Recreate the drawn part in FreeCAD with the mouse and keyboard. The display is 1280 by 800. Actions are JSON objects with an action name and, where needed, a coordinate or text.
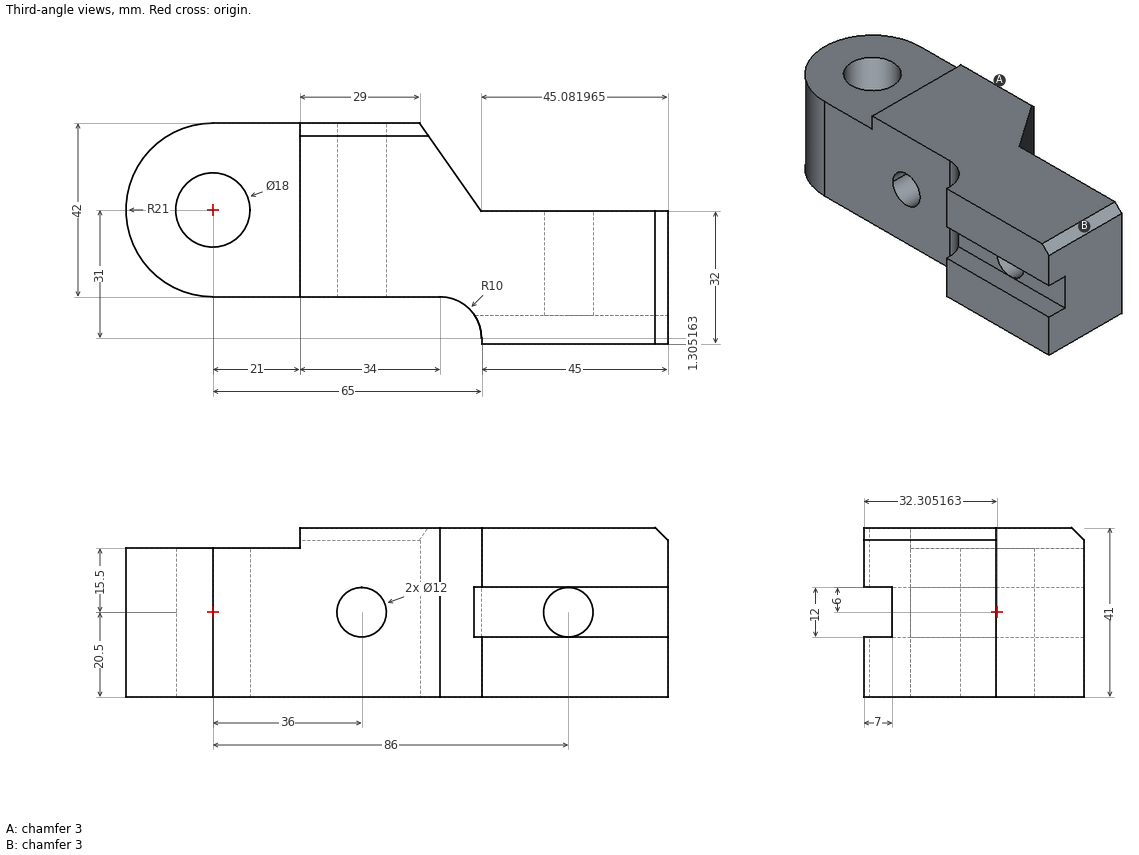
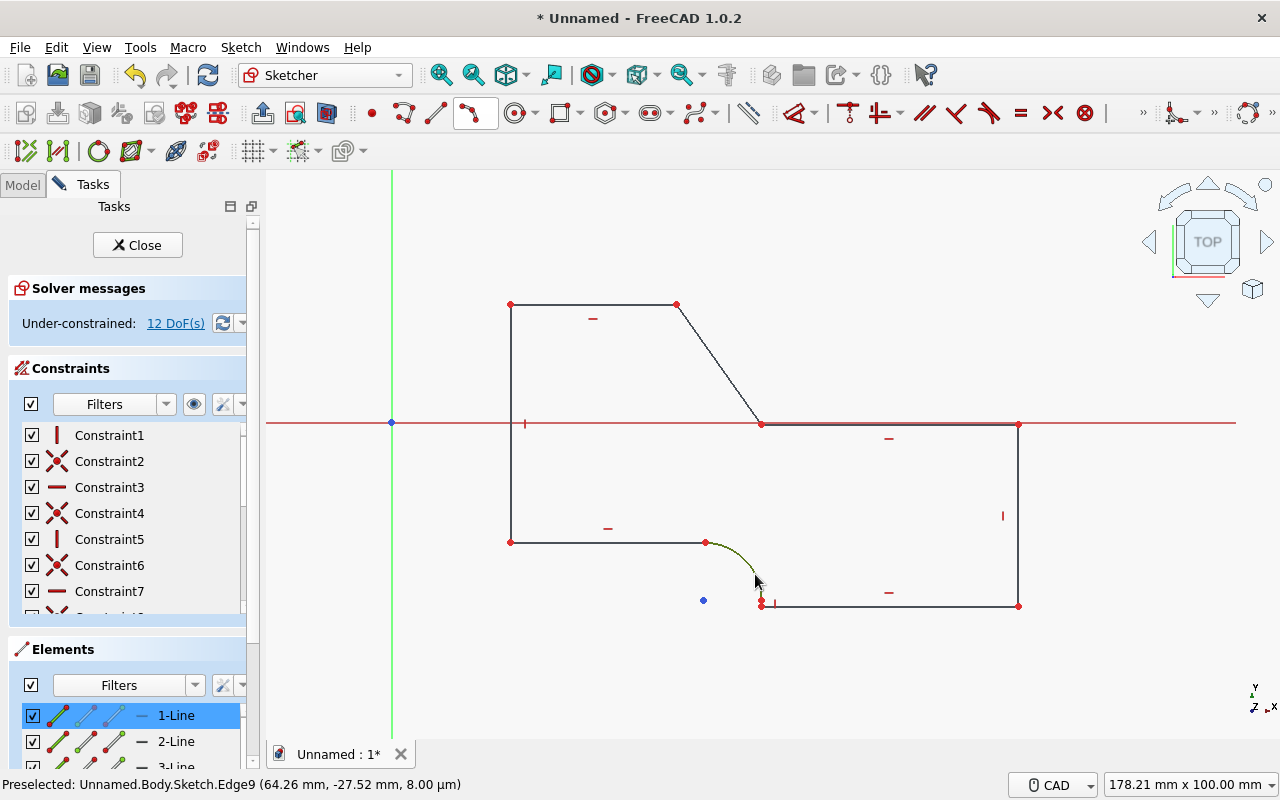
{"action": "left_click", "coordinate": [990, 114]}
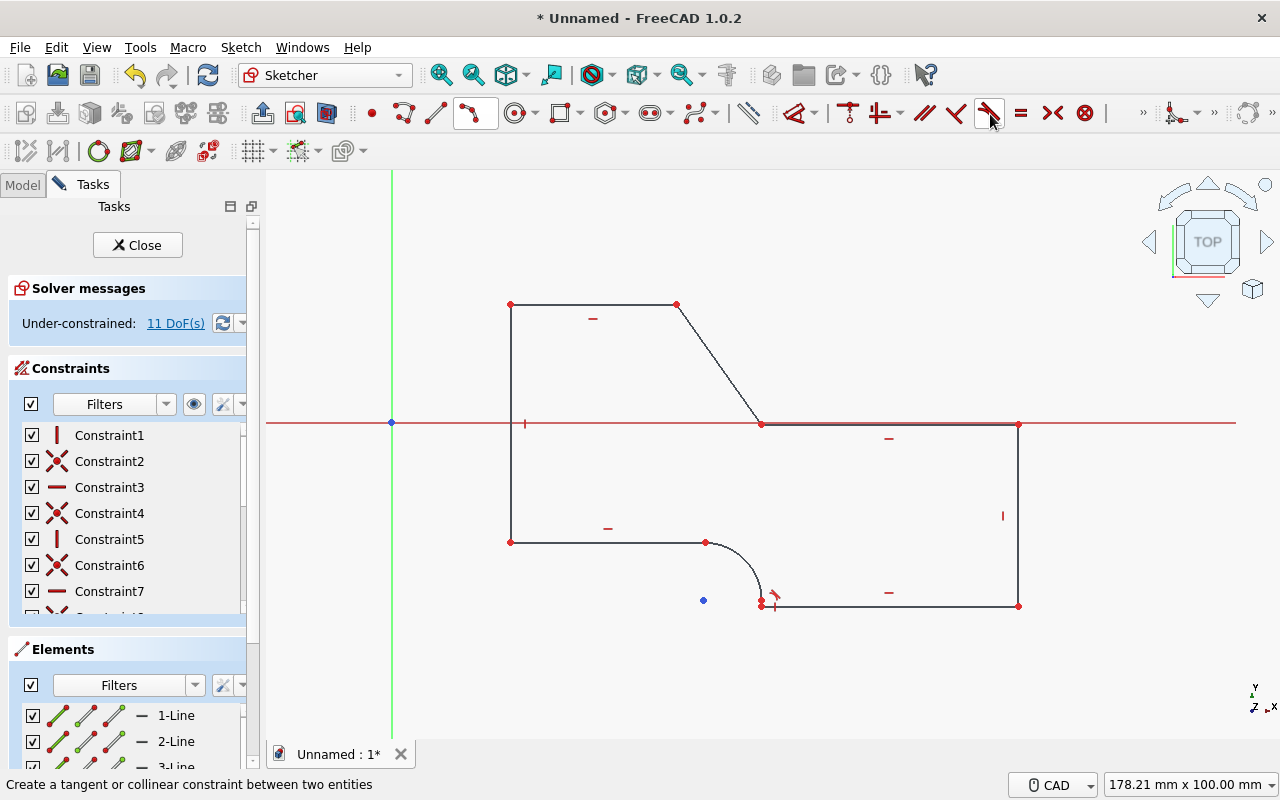
{"action": "left_click", "coordinate": [569, 543]}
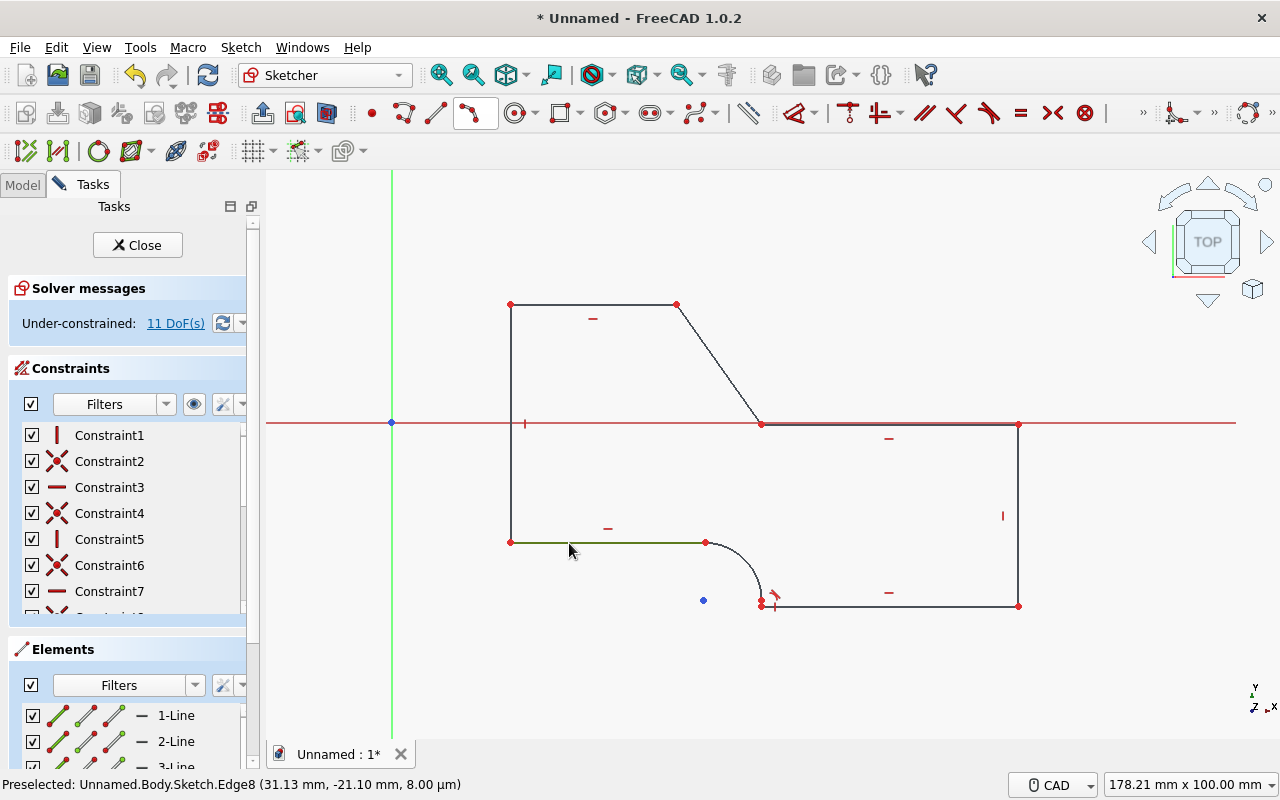
{"action": "left_click", "coordinate": [755, 575]}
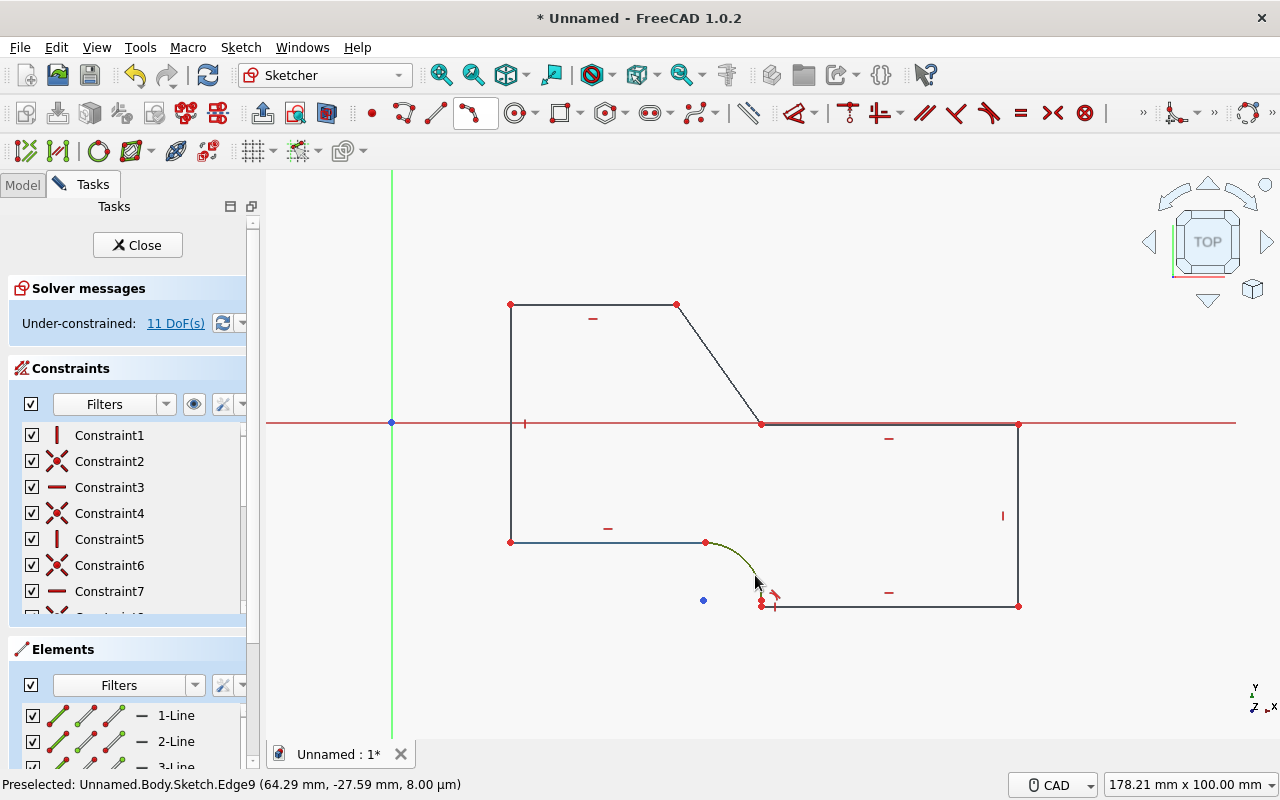
{"action": "left_click", "coordinate": [990, 114]}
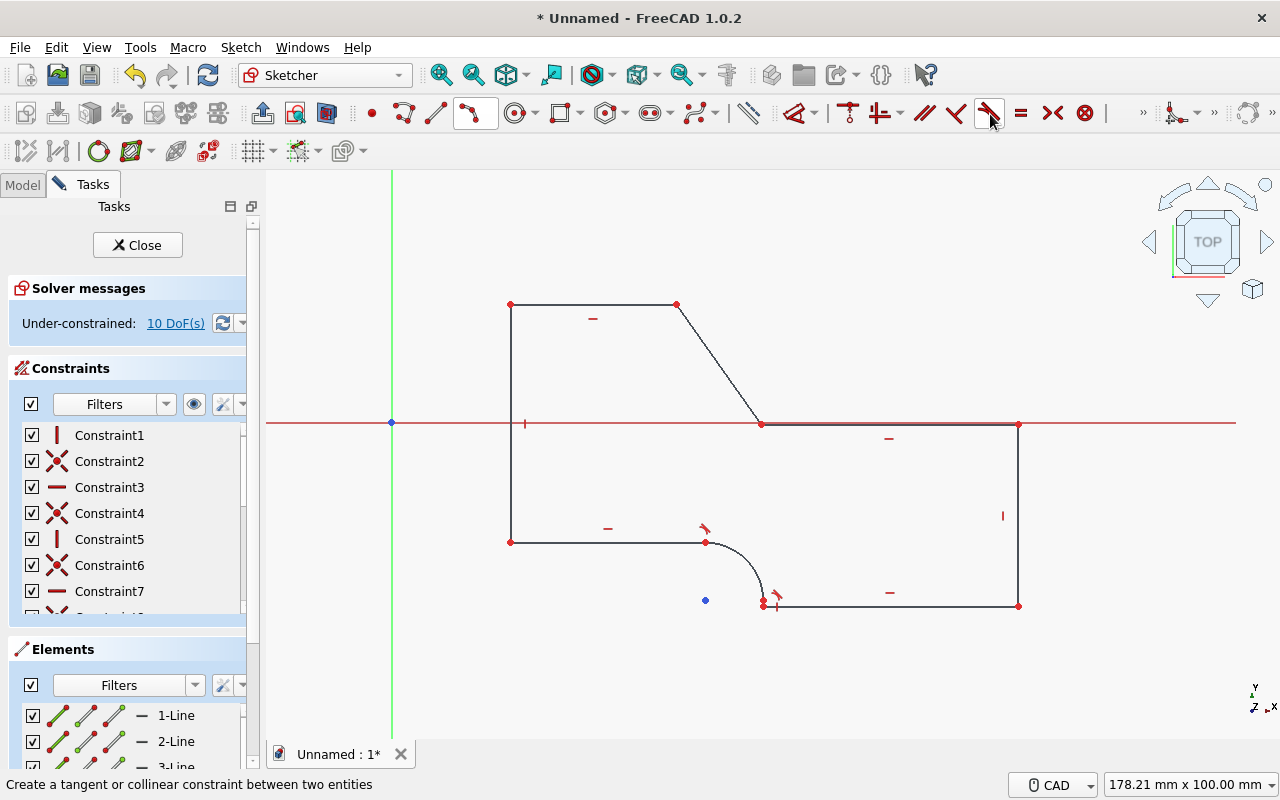
{"action": "left_click", "coordinate": [794, 114]}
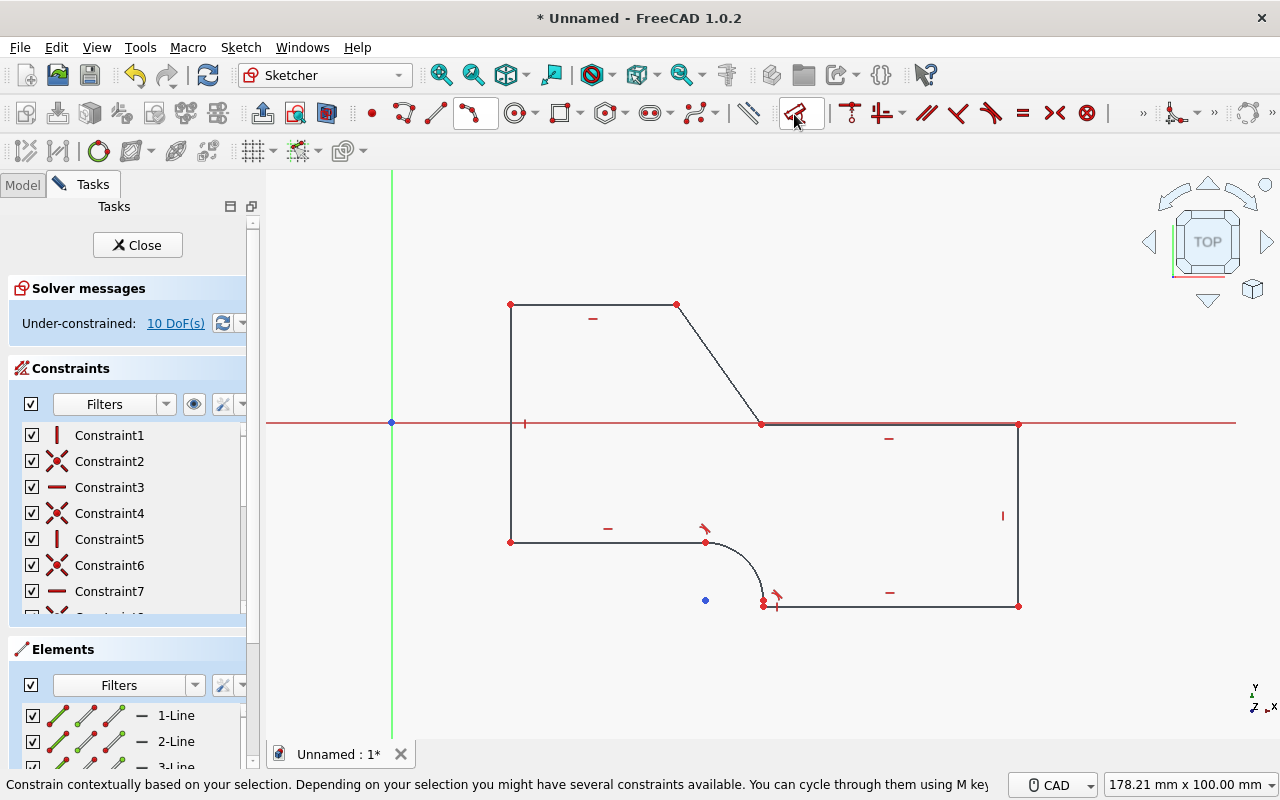
{"action": "left_click", "coordinate": [757, 574]}
{"action": "left_click", "coordinate": [785, 559]}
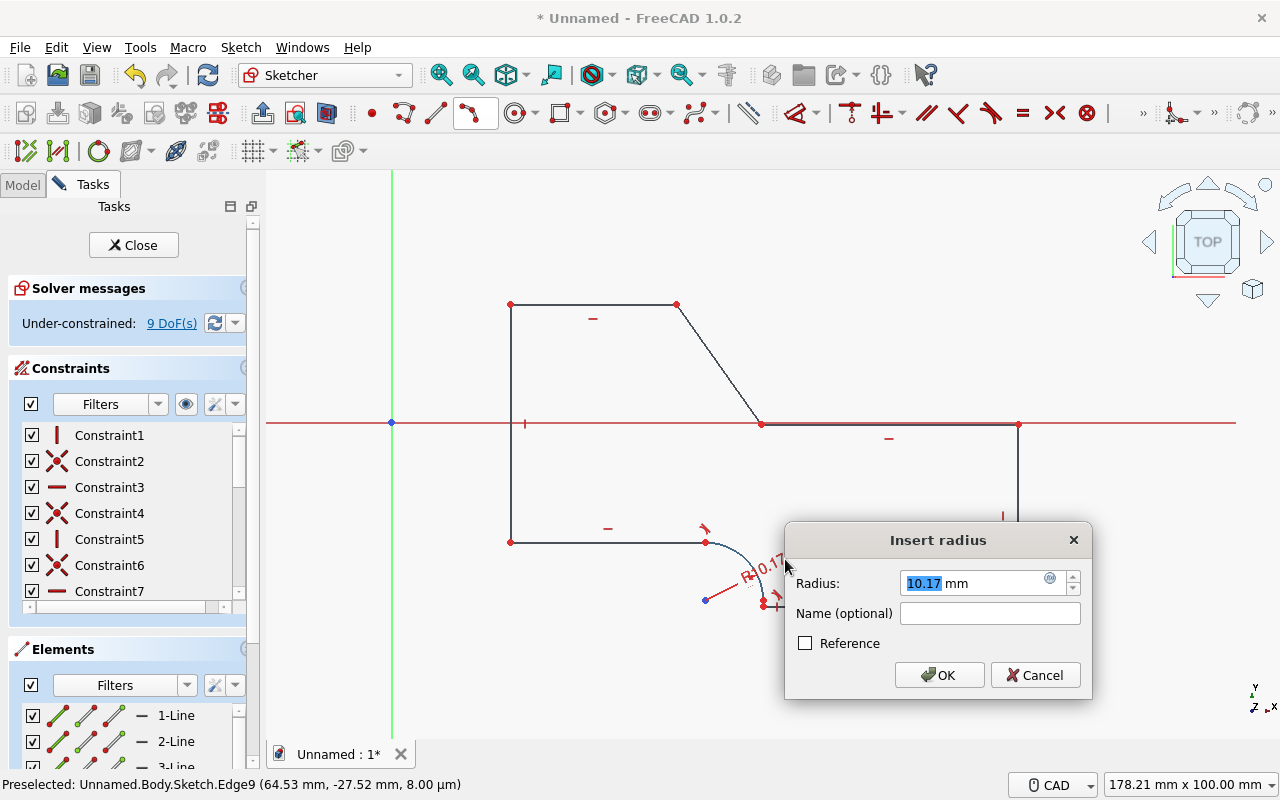
{"action": "type", "text": "10"}
{"action": "key", "text": "Return"}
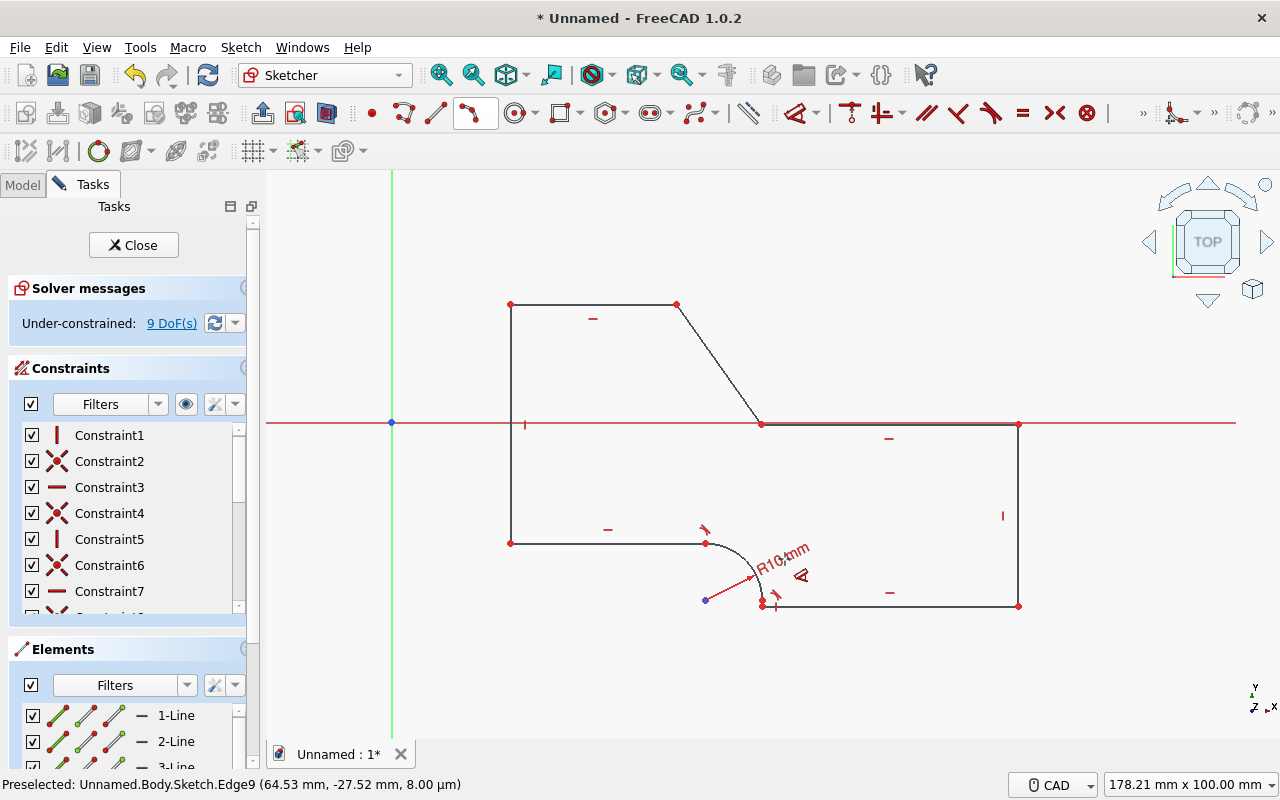
{"action": "left_click", "coordinate": [839, 607]}
{"action": "left_click", "coordinate": [890, 641]}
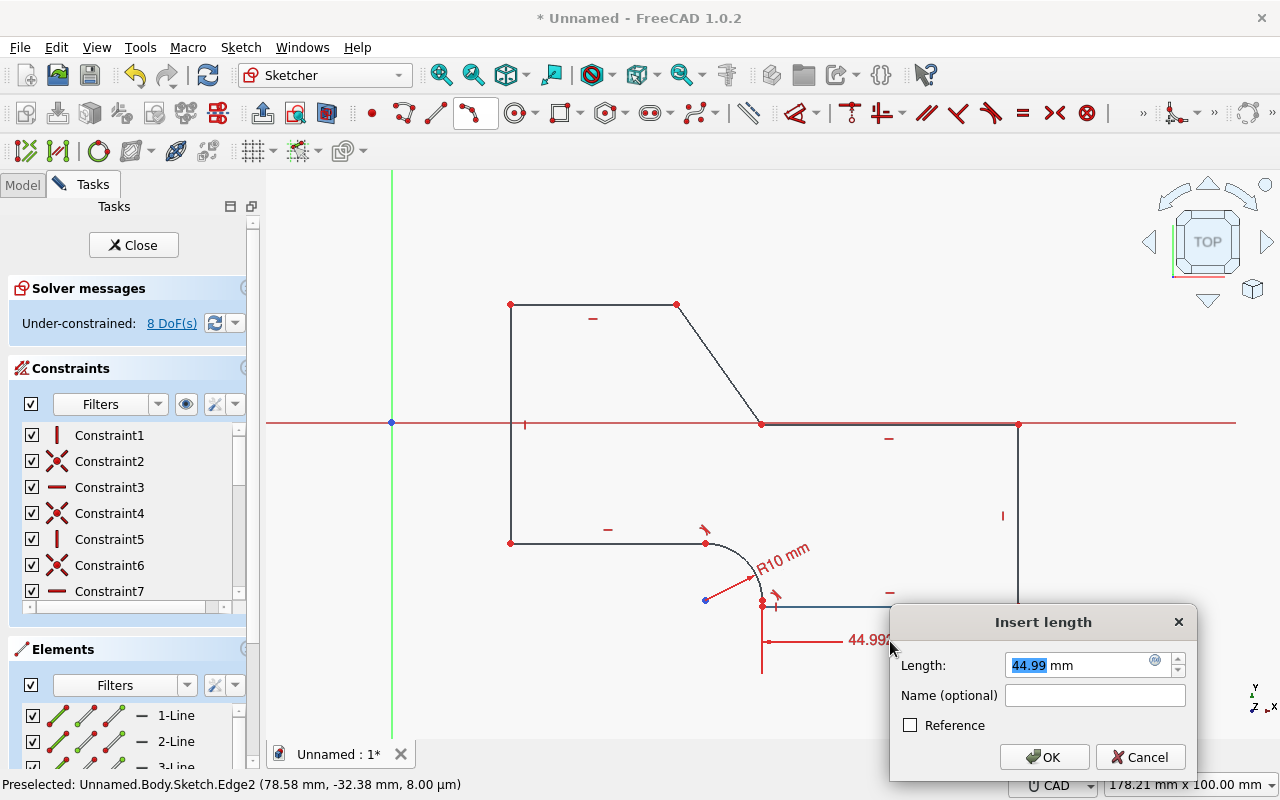
{"action": "type", "text": "45"}
{"action": "key", "text": "Return"}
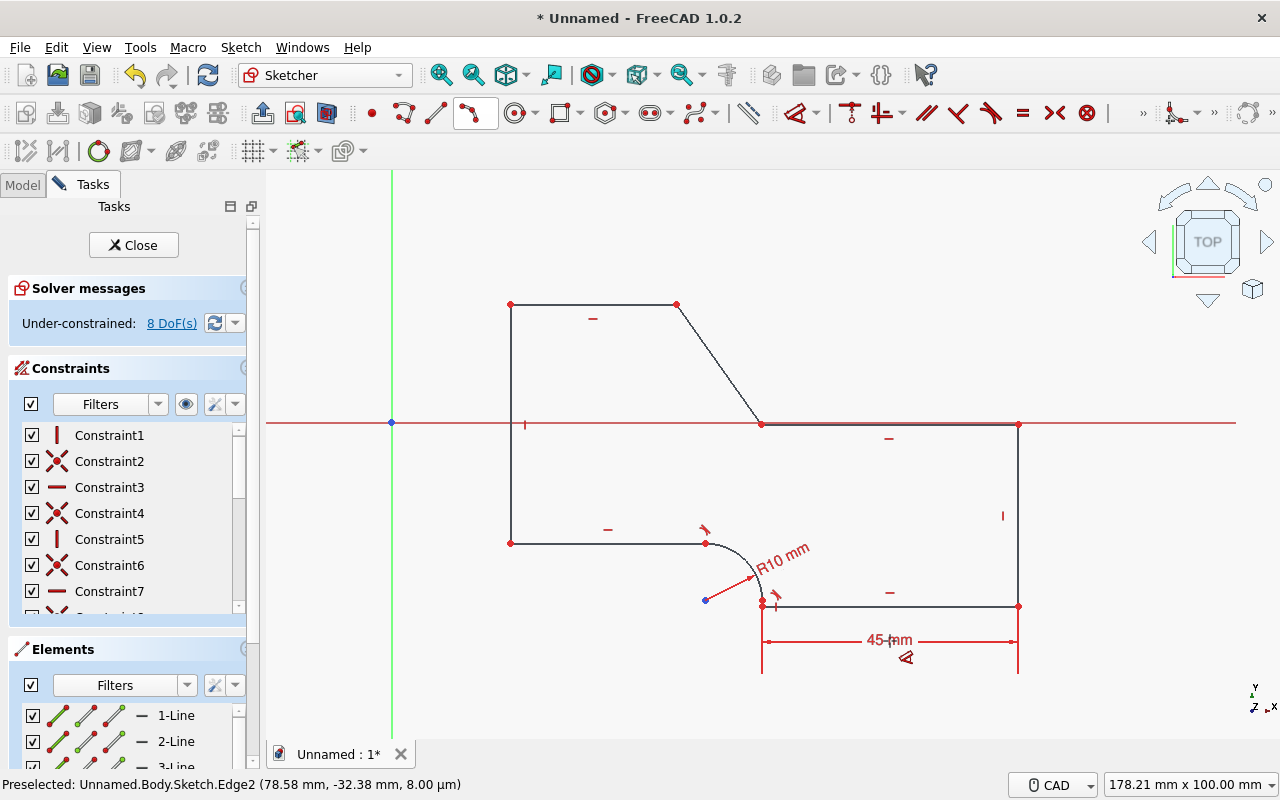
{"action": "left_click", "coordinate": [1018, 552]}
{"action": "left_click", "coordinate": [1052, 516]}